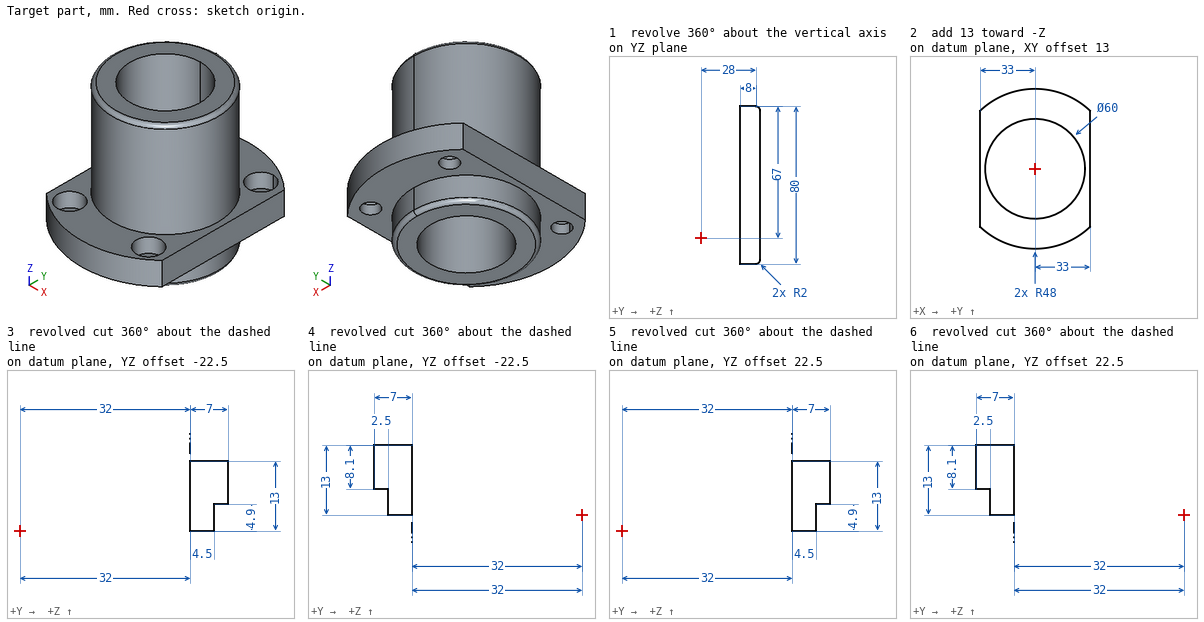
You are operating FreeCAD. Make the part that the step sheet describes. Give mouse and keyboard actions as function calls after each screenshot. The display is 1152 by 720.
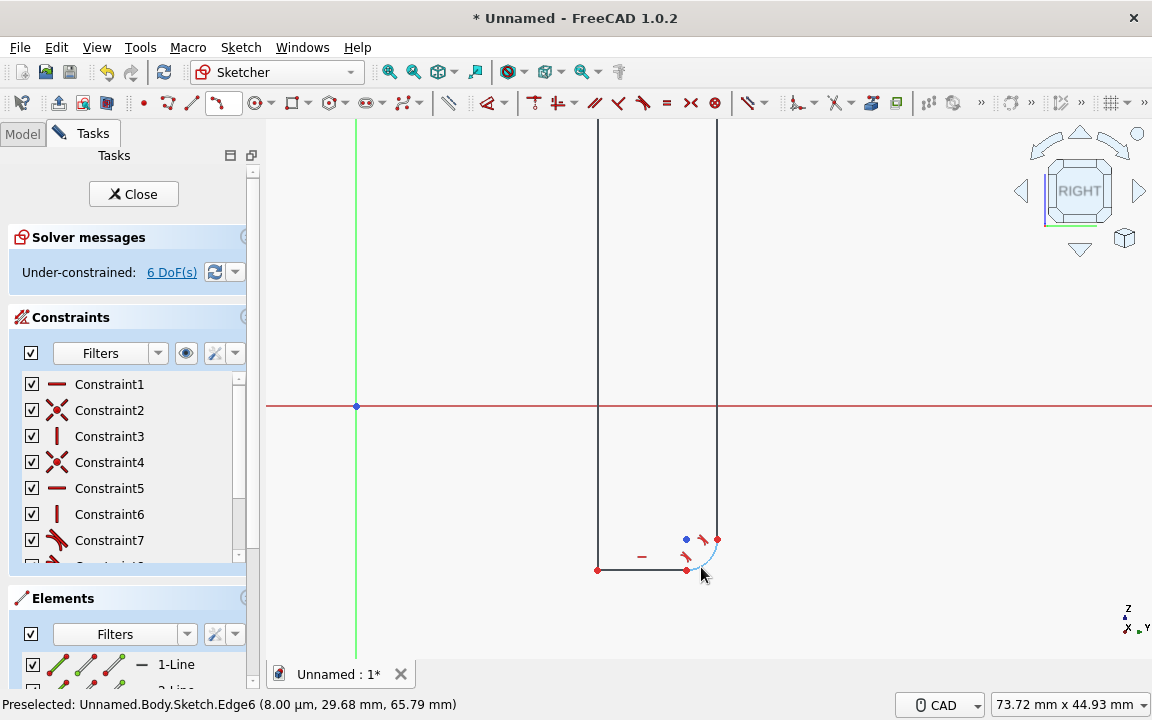
click(700, 567)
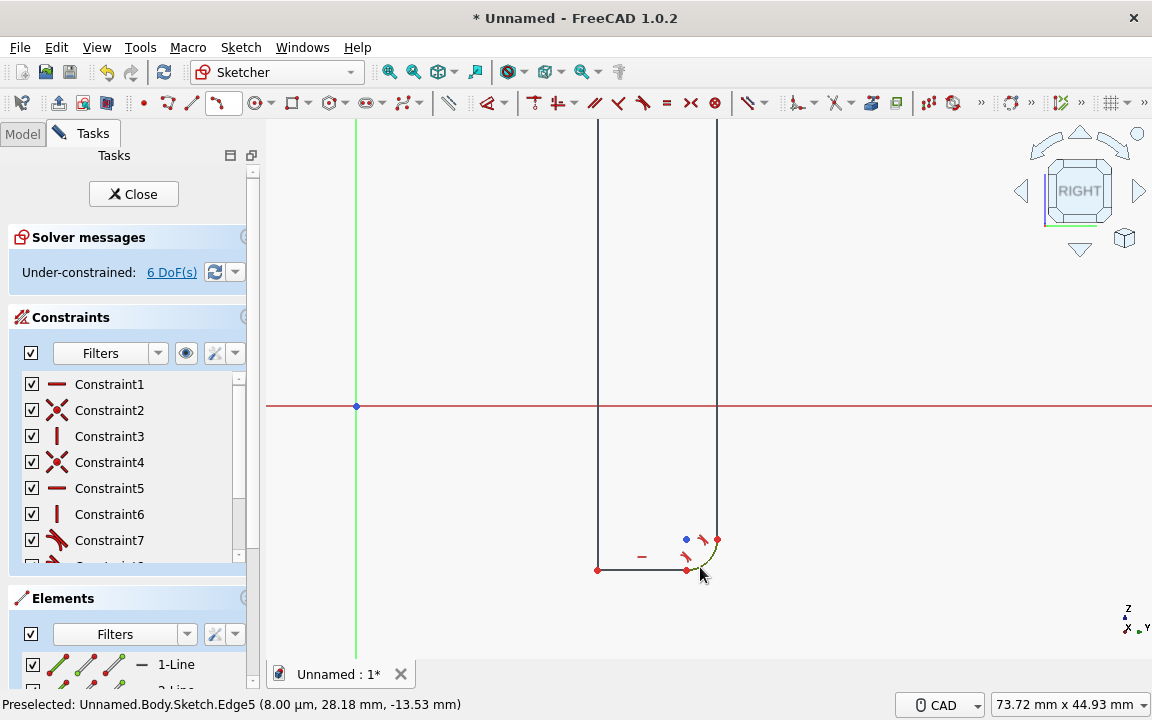
scroll(701, 568, down, 5)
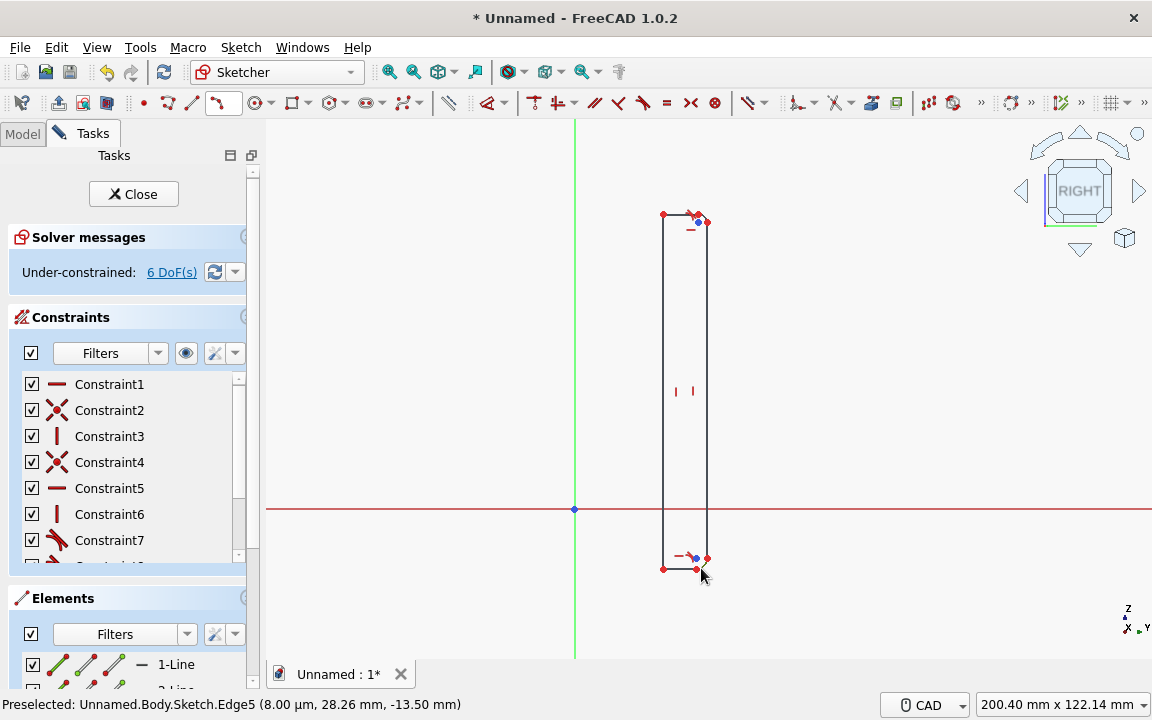
scroll(706, 219, up, 7)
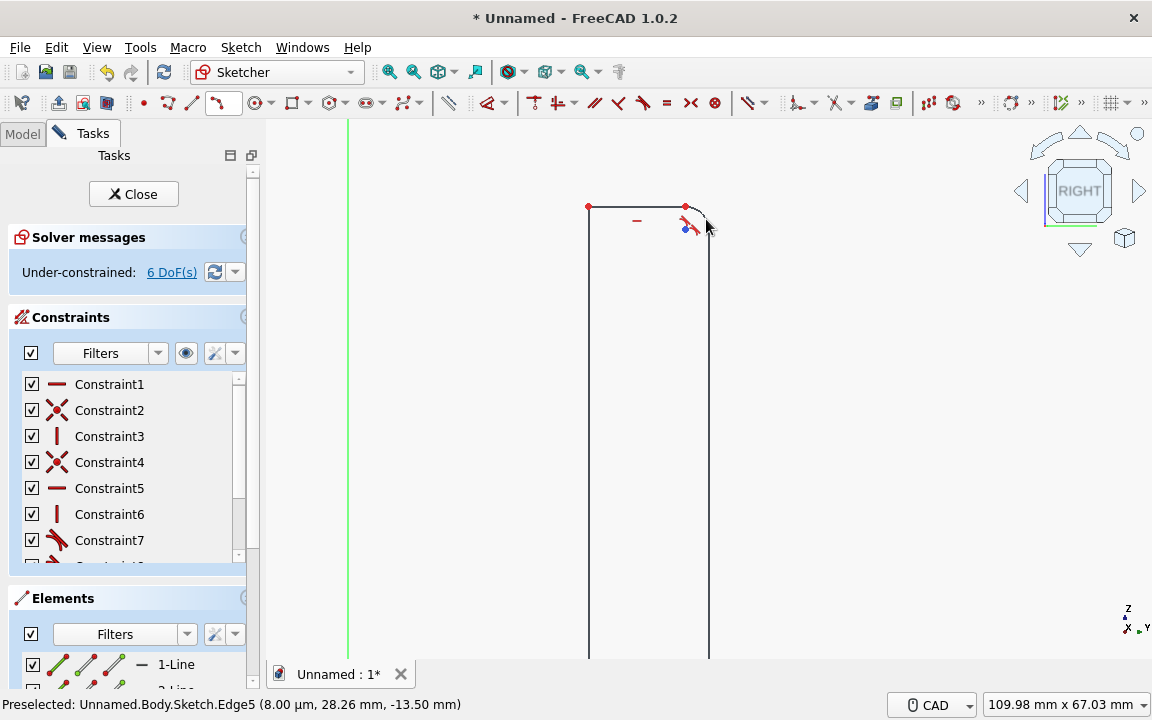
click(706, 219)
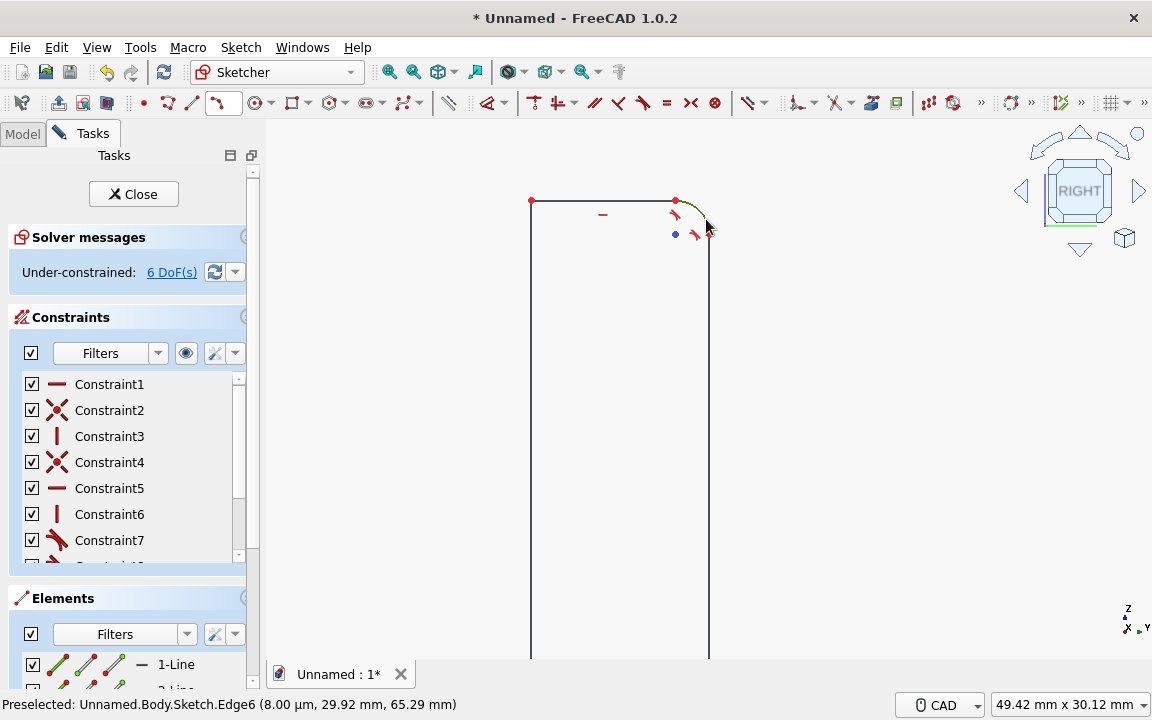
click(668, 104)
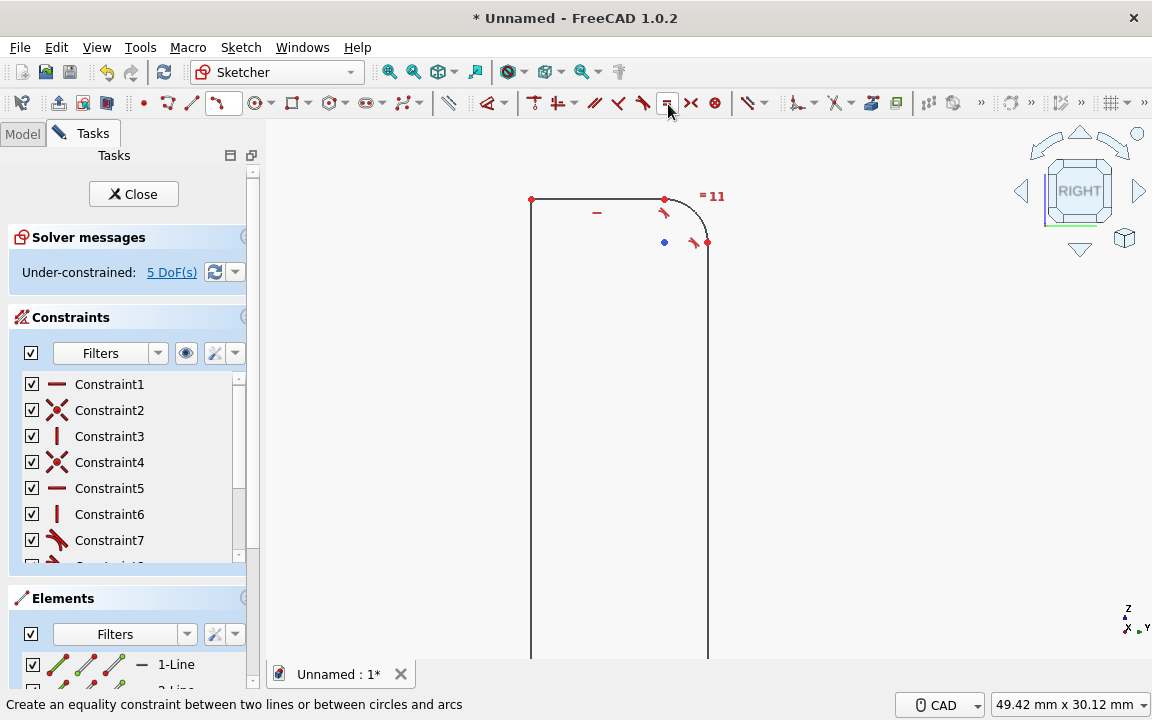
scroll(706, 218, down, 7)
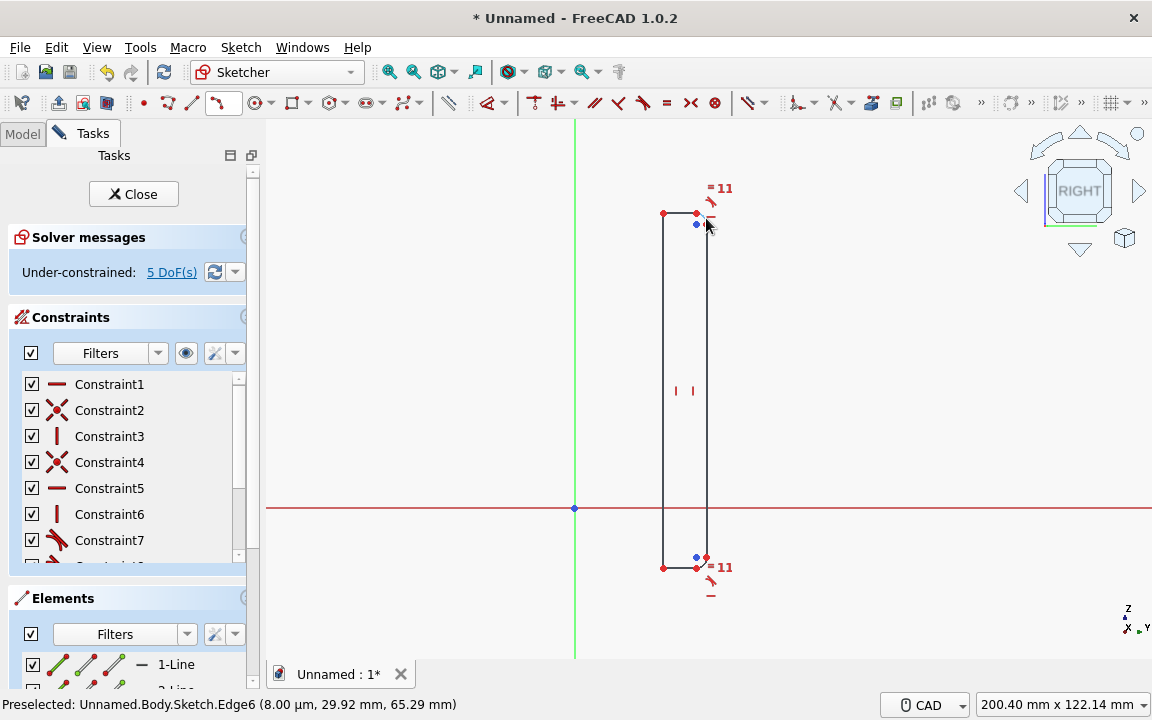
scroll(701, 567, up, 8)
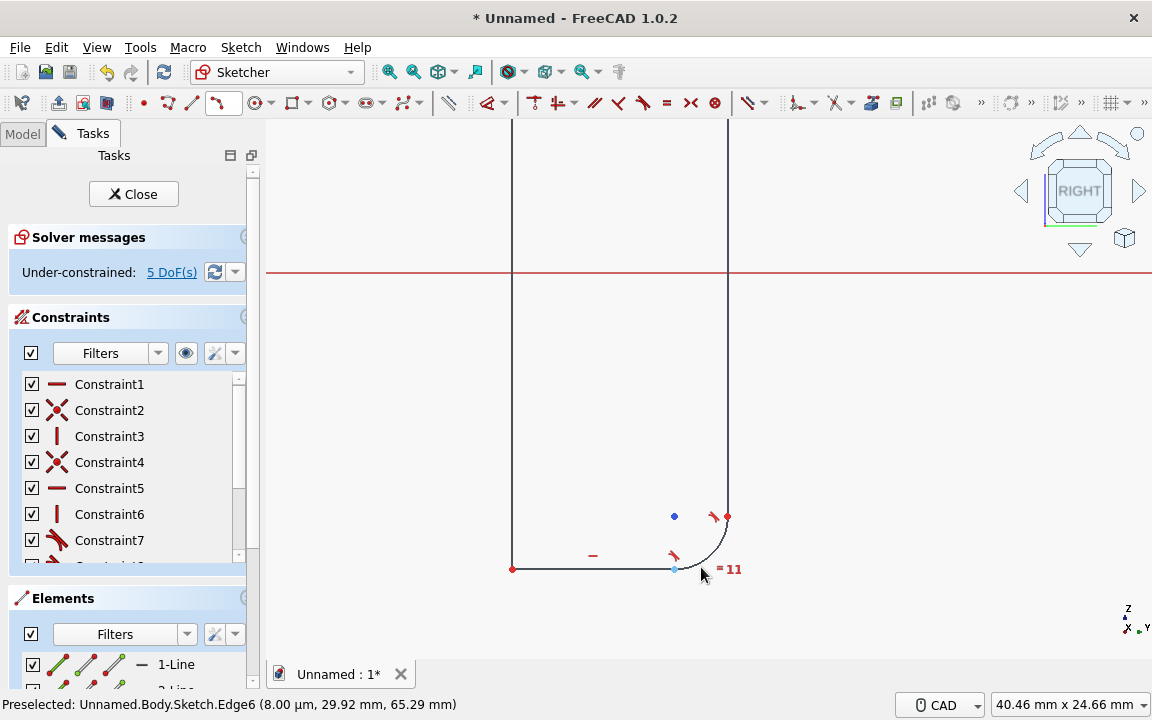
click(699, 564)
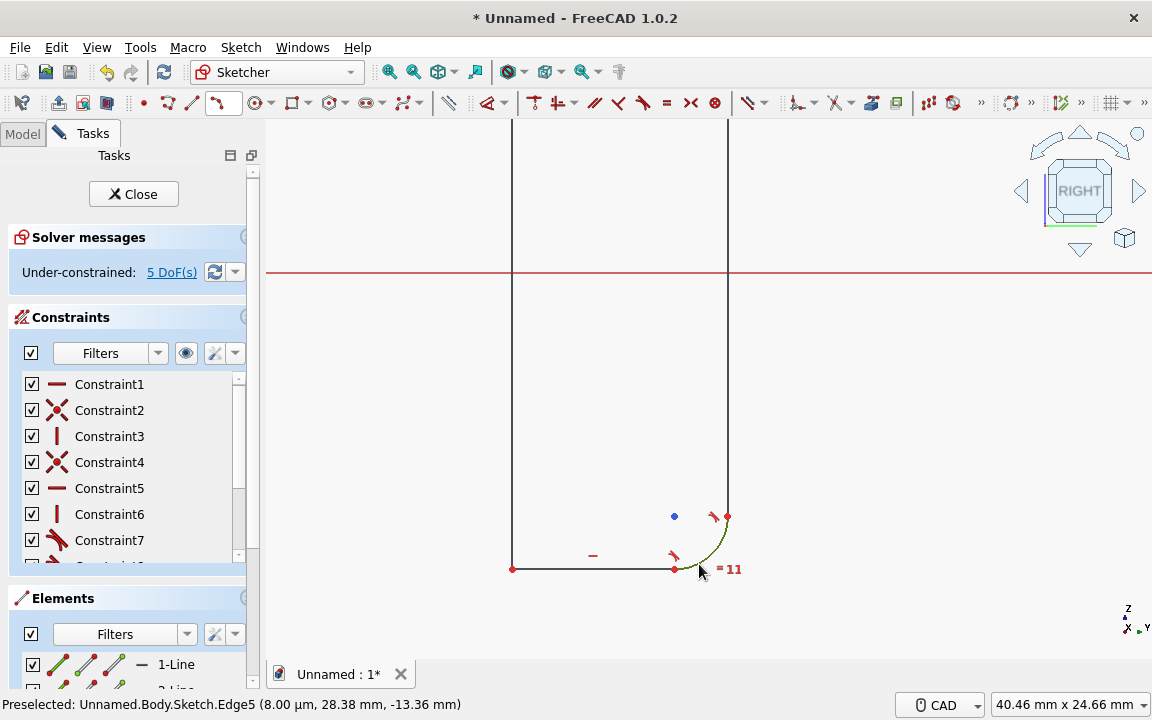
click(506, 104)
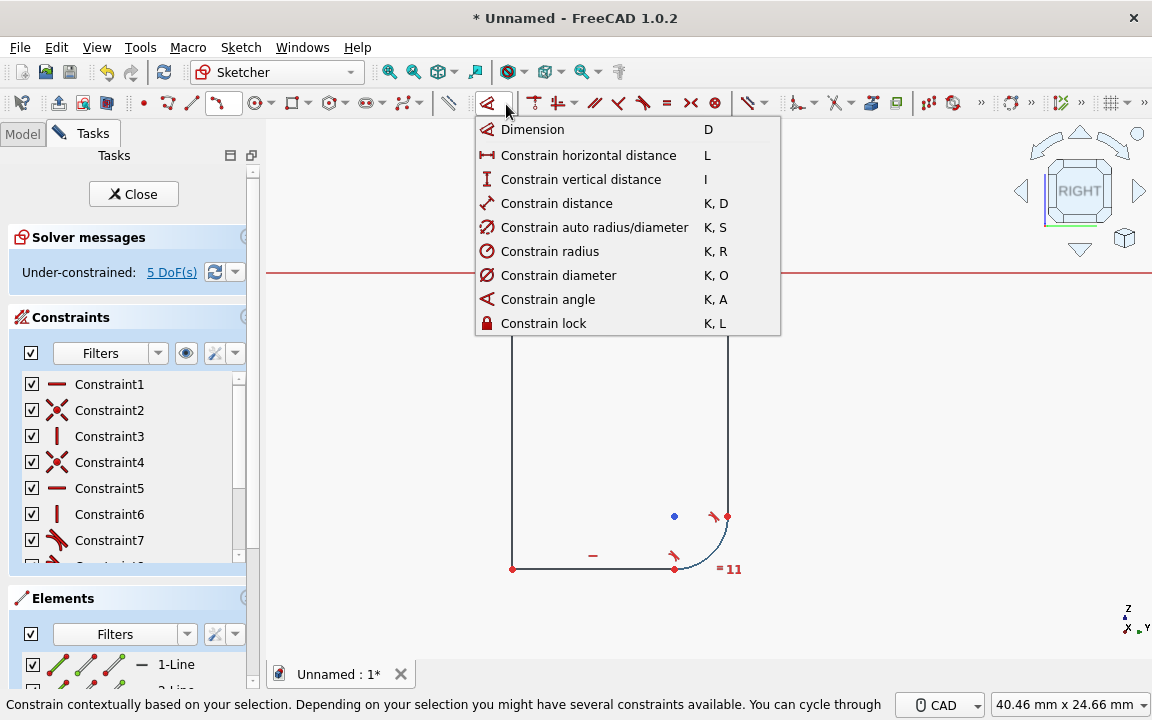
click(628, 251)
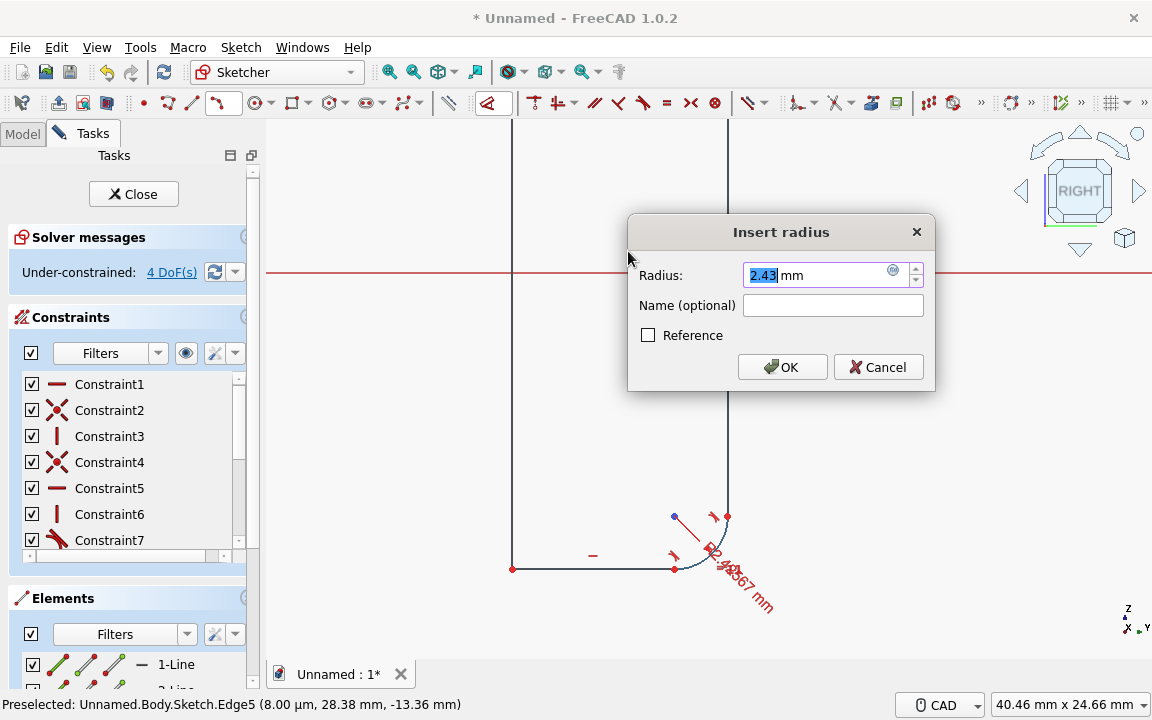
text(2)
key(Return)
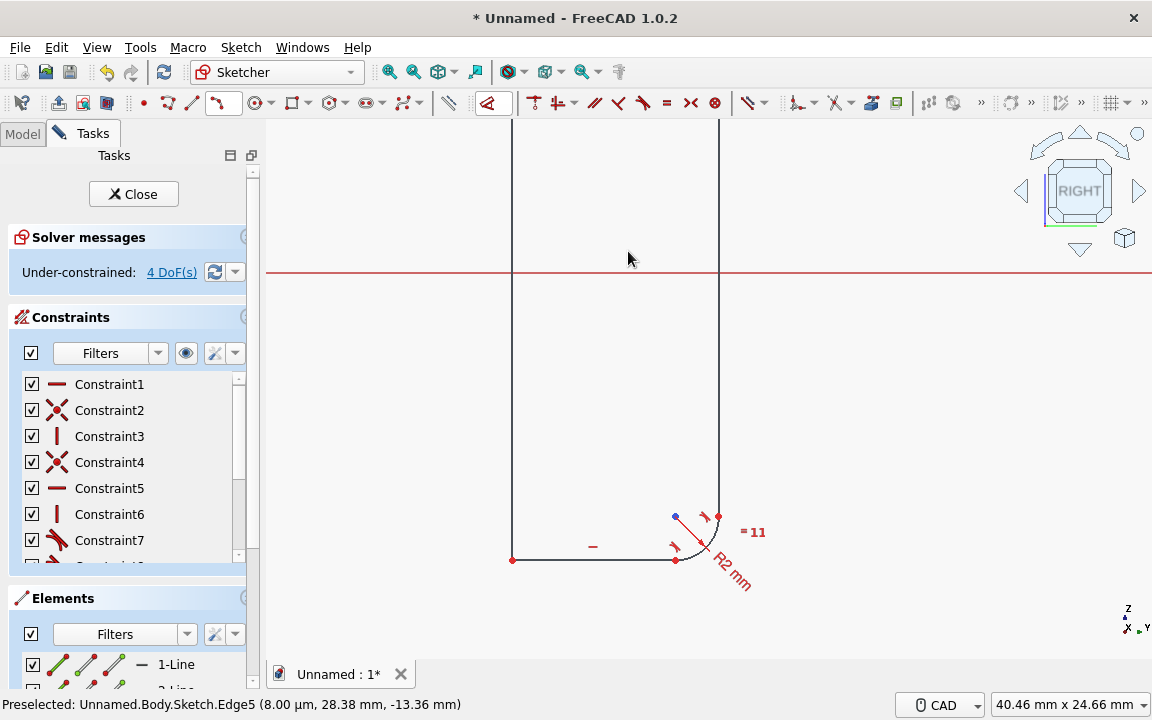
scroll(701, 568, down, 8)